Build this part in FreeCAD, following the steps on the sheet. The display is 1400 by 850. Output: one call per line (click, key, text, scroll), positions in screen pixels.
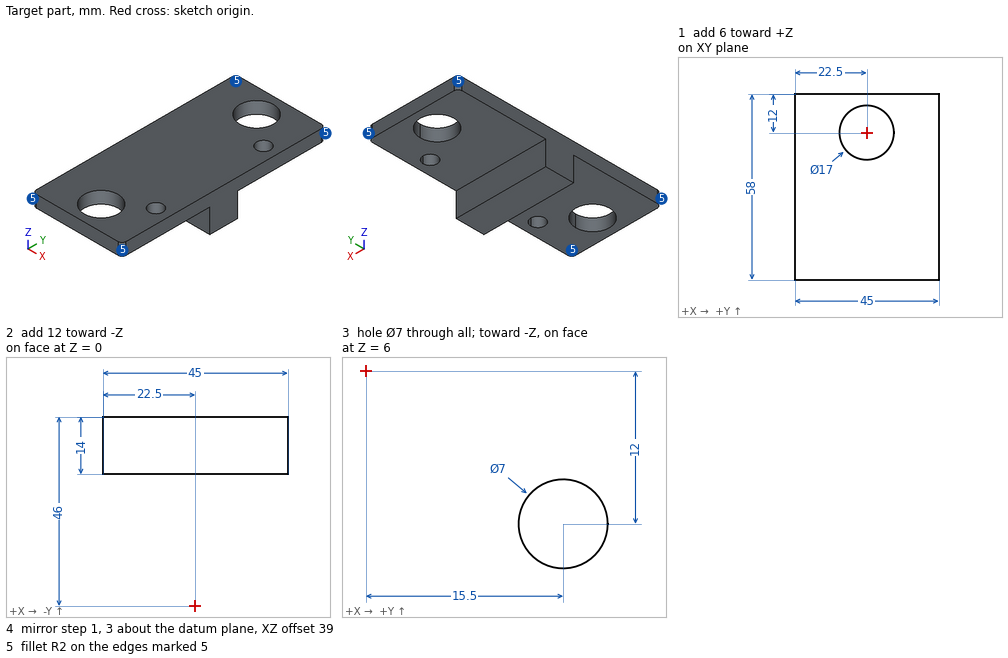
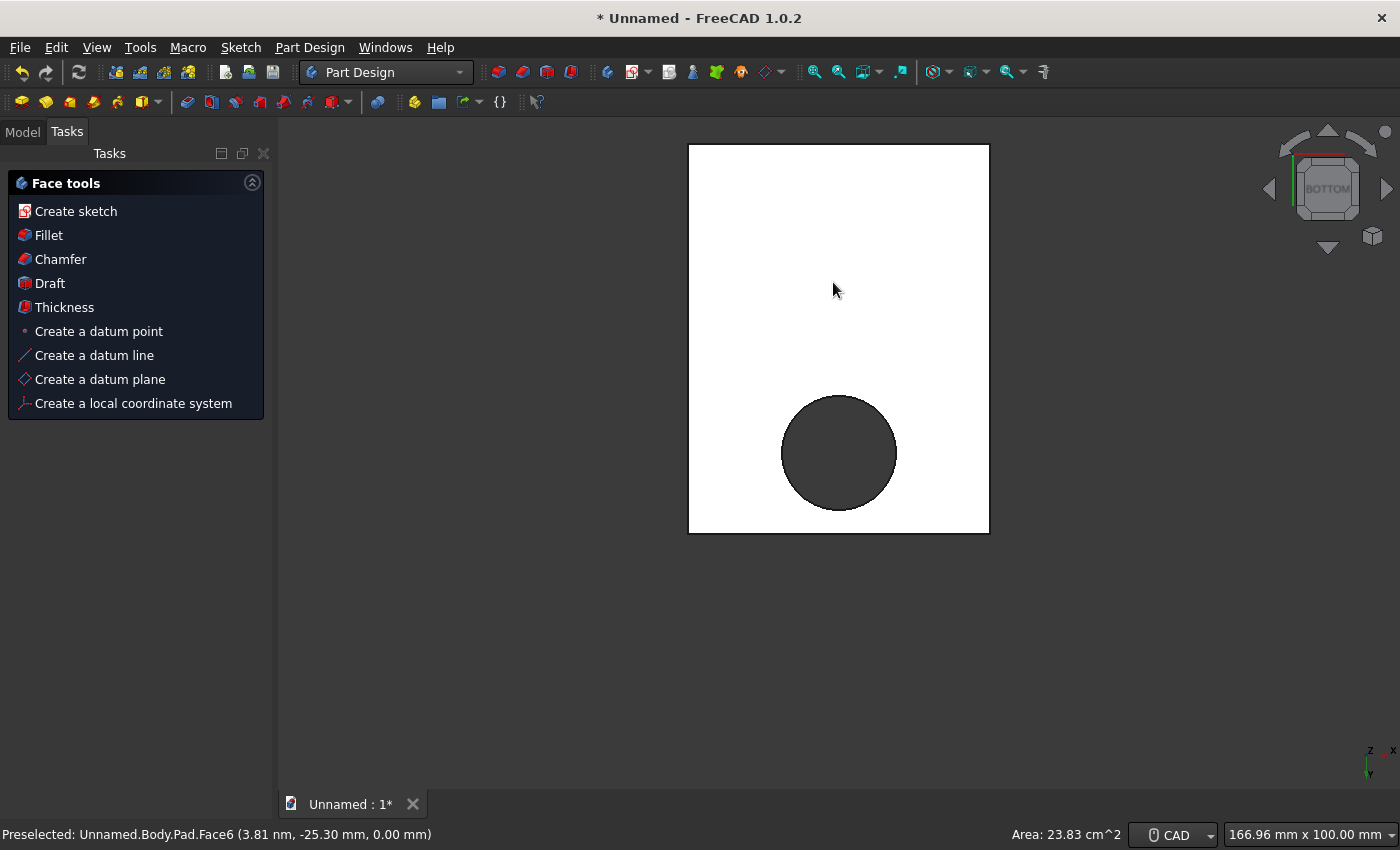
click(632, 72)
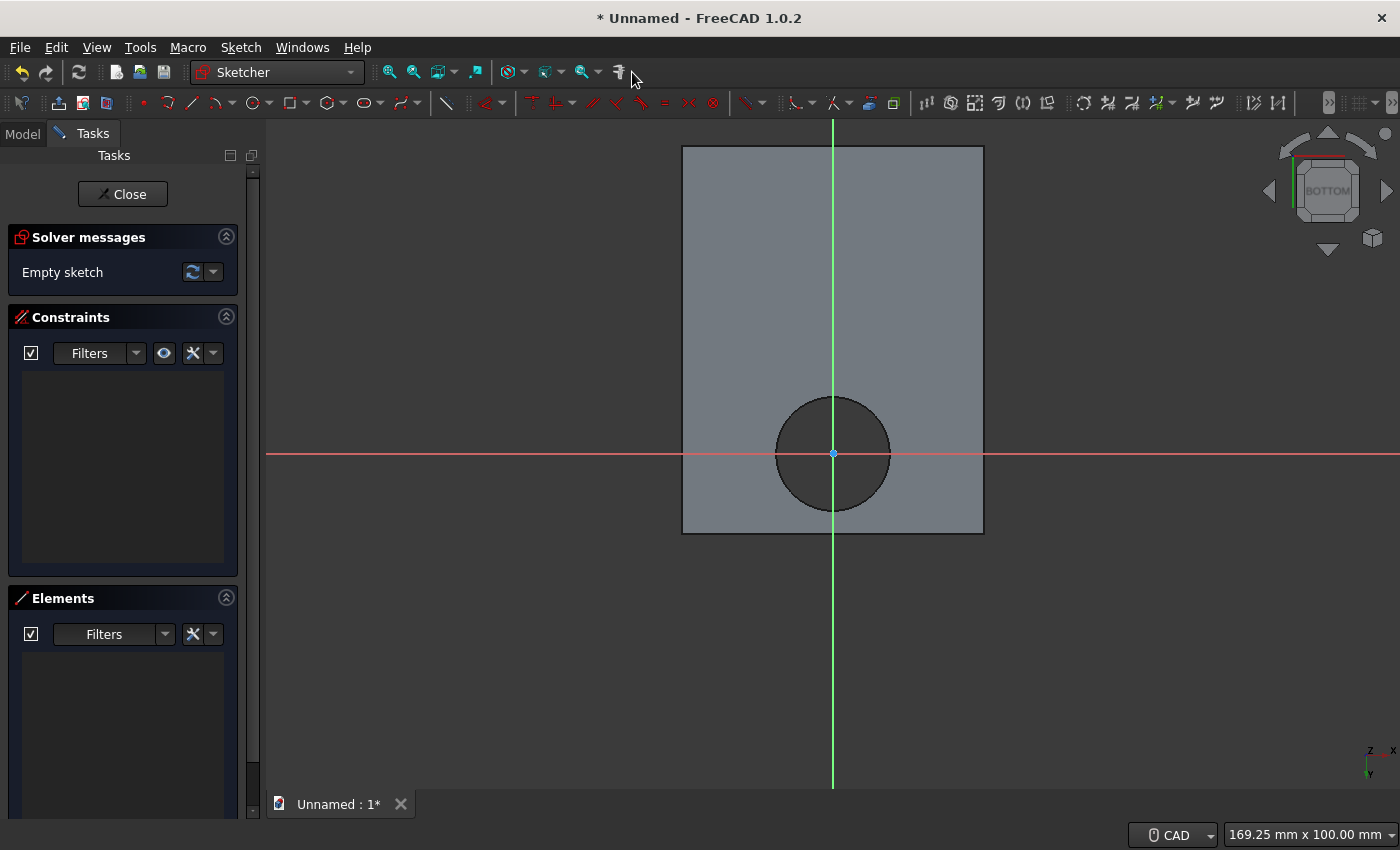
scroll(455, 761, down, 1)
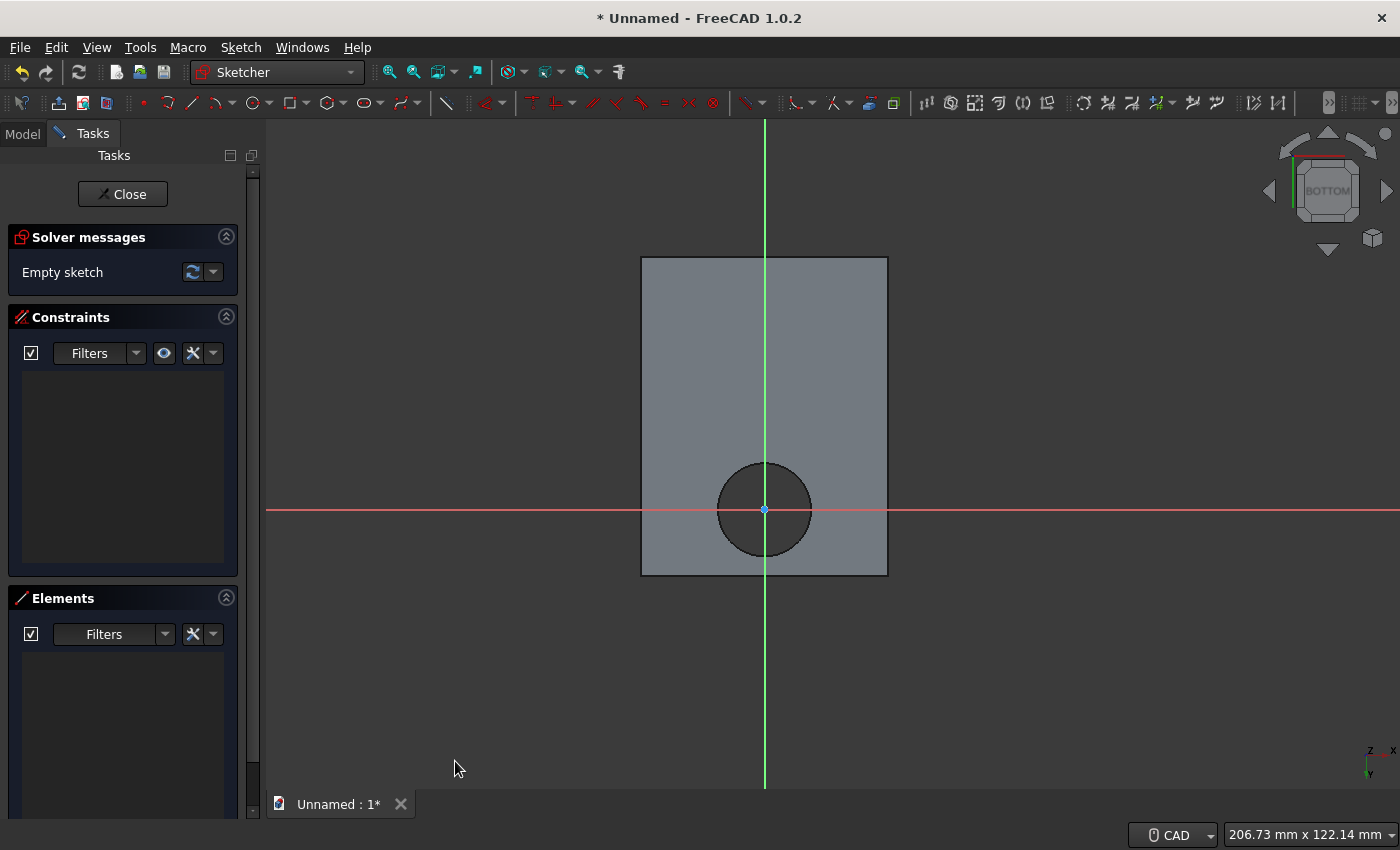
scroll(765, 298, up, 3)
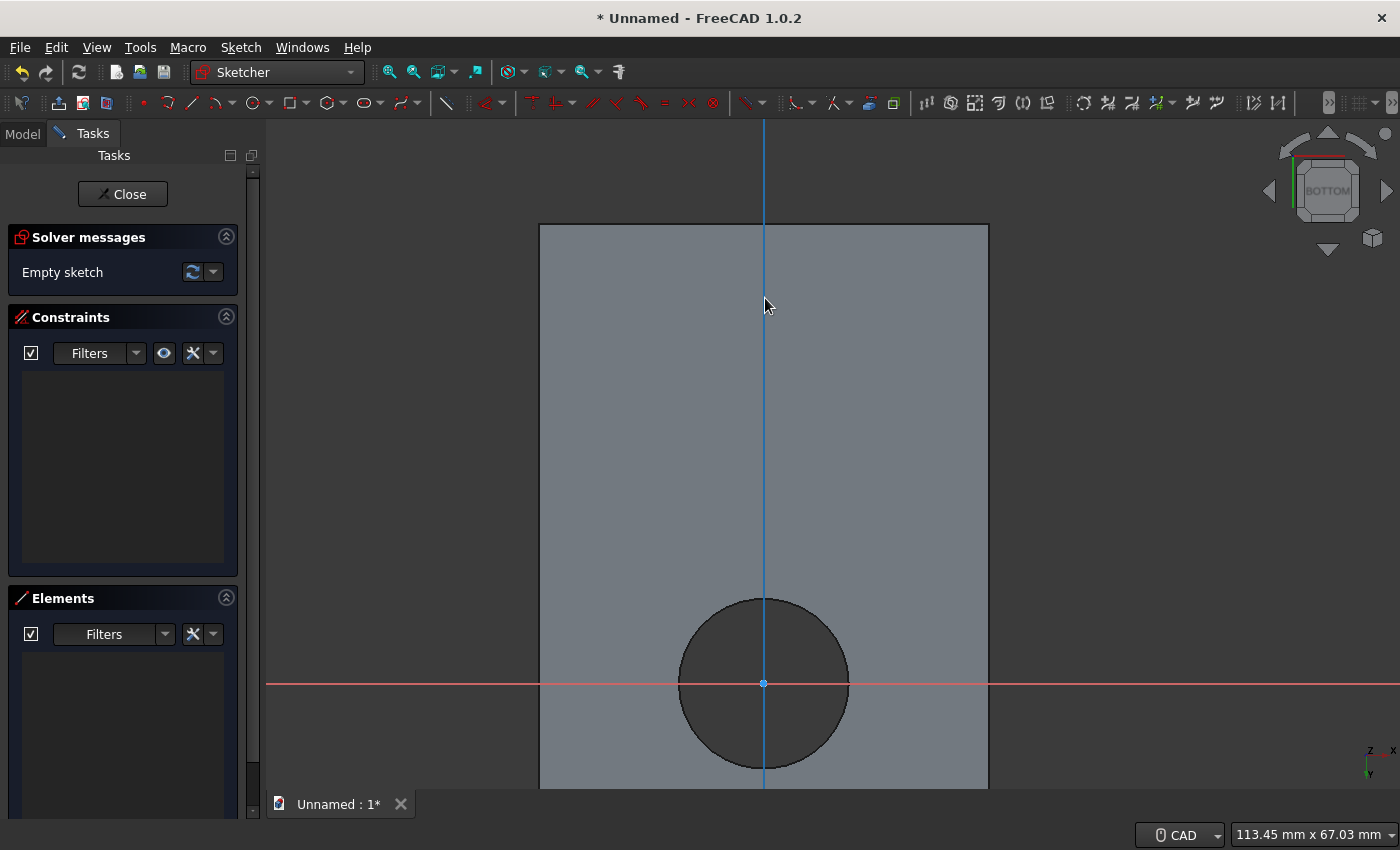
click(290, 104)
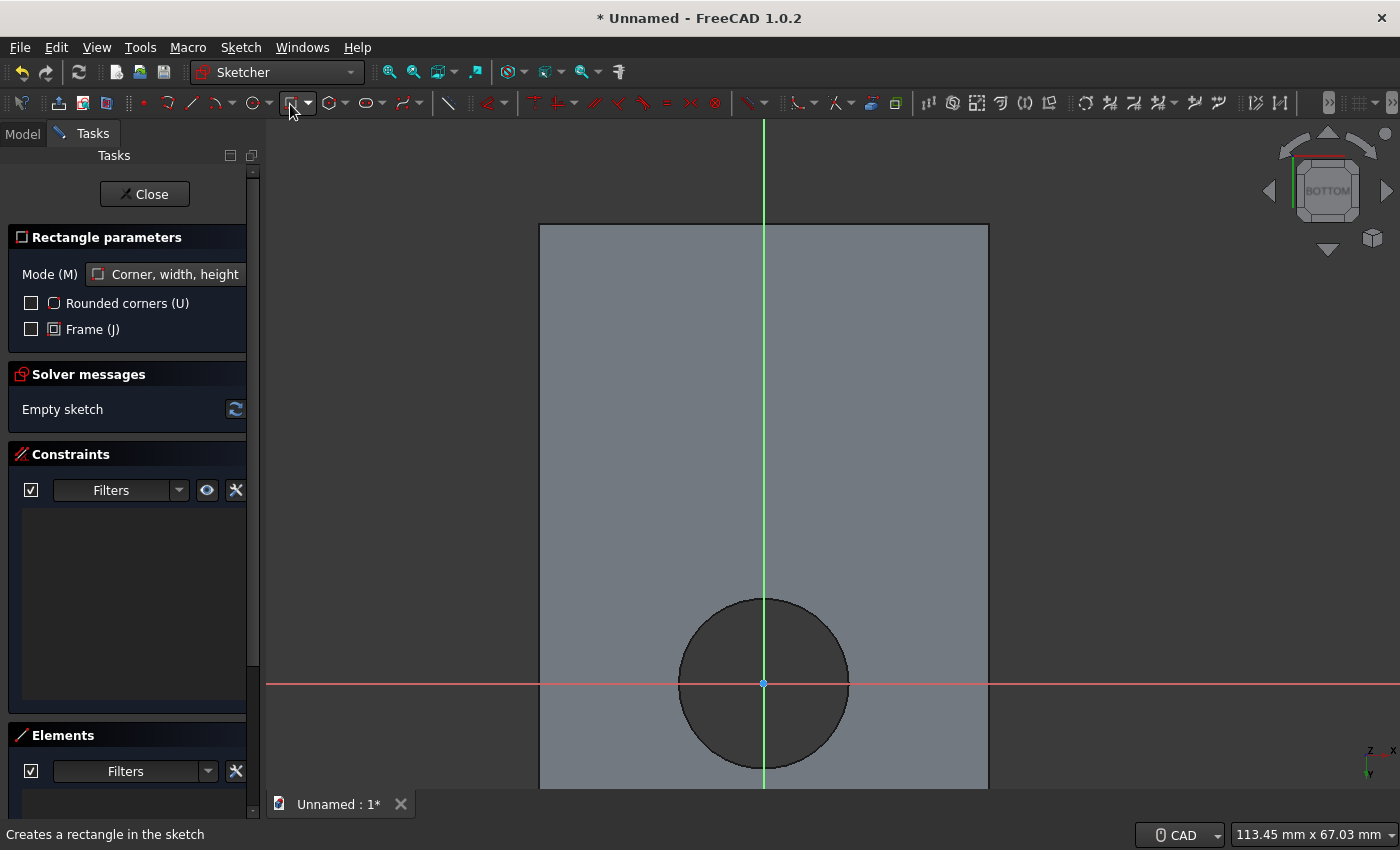
click(539, 224)
click(989, 364)
key(Escape)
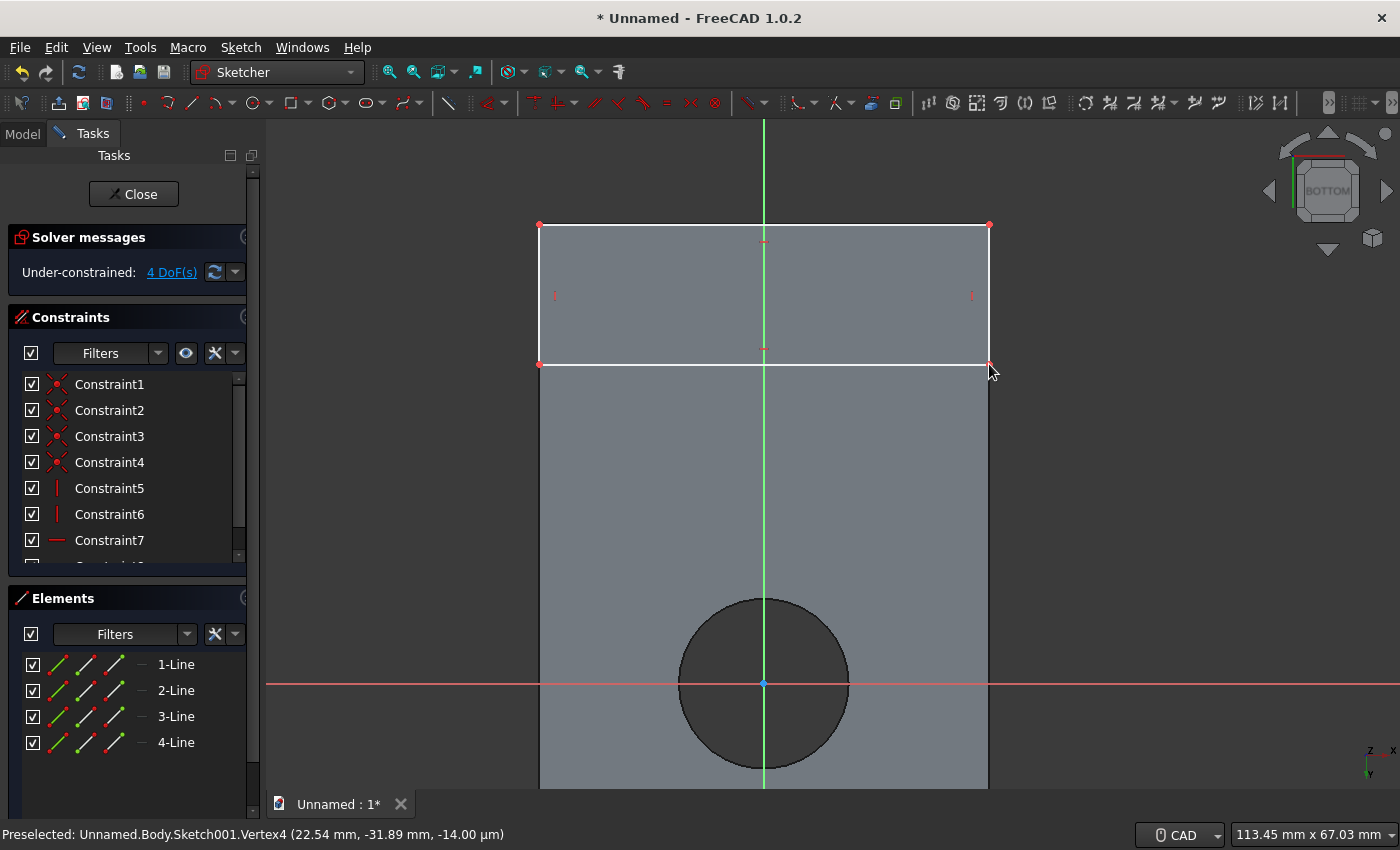
click(488, 104)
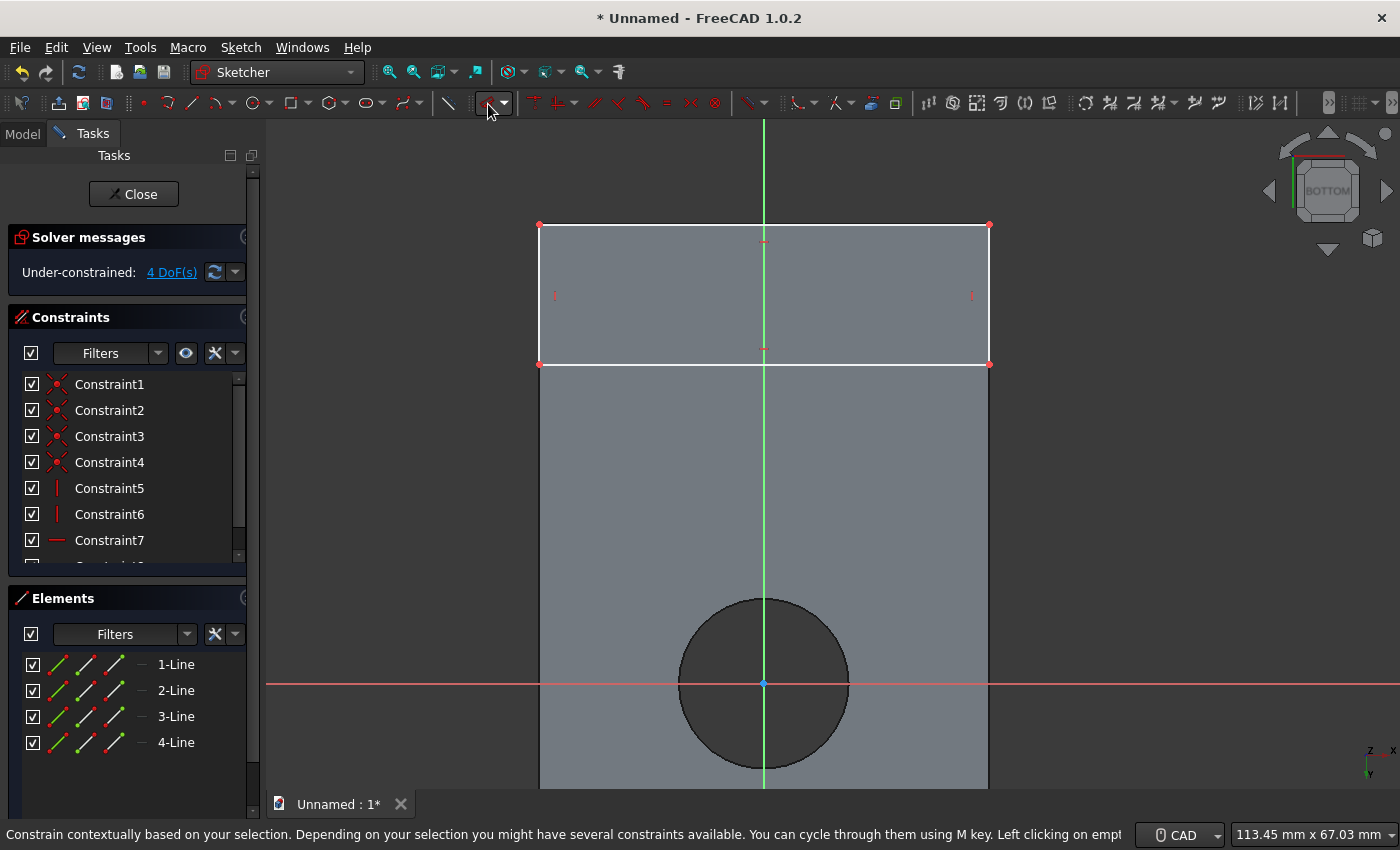
click(539, 267)
click(505, 295)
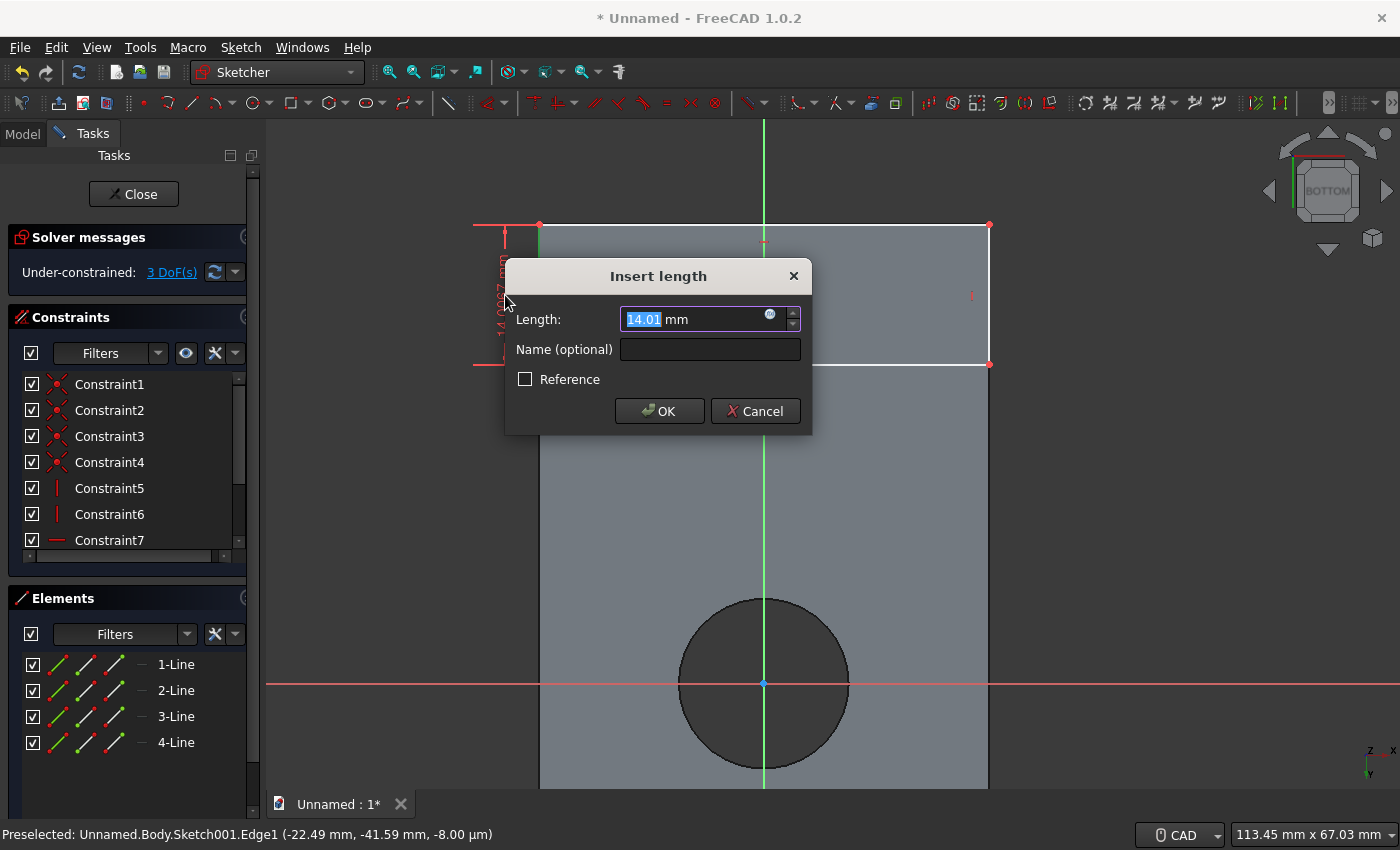
text(14)
key(Return)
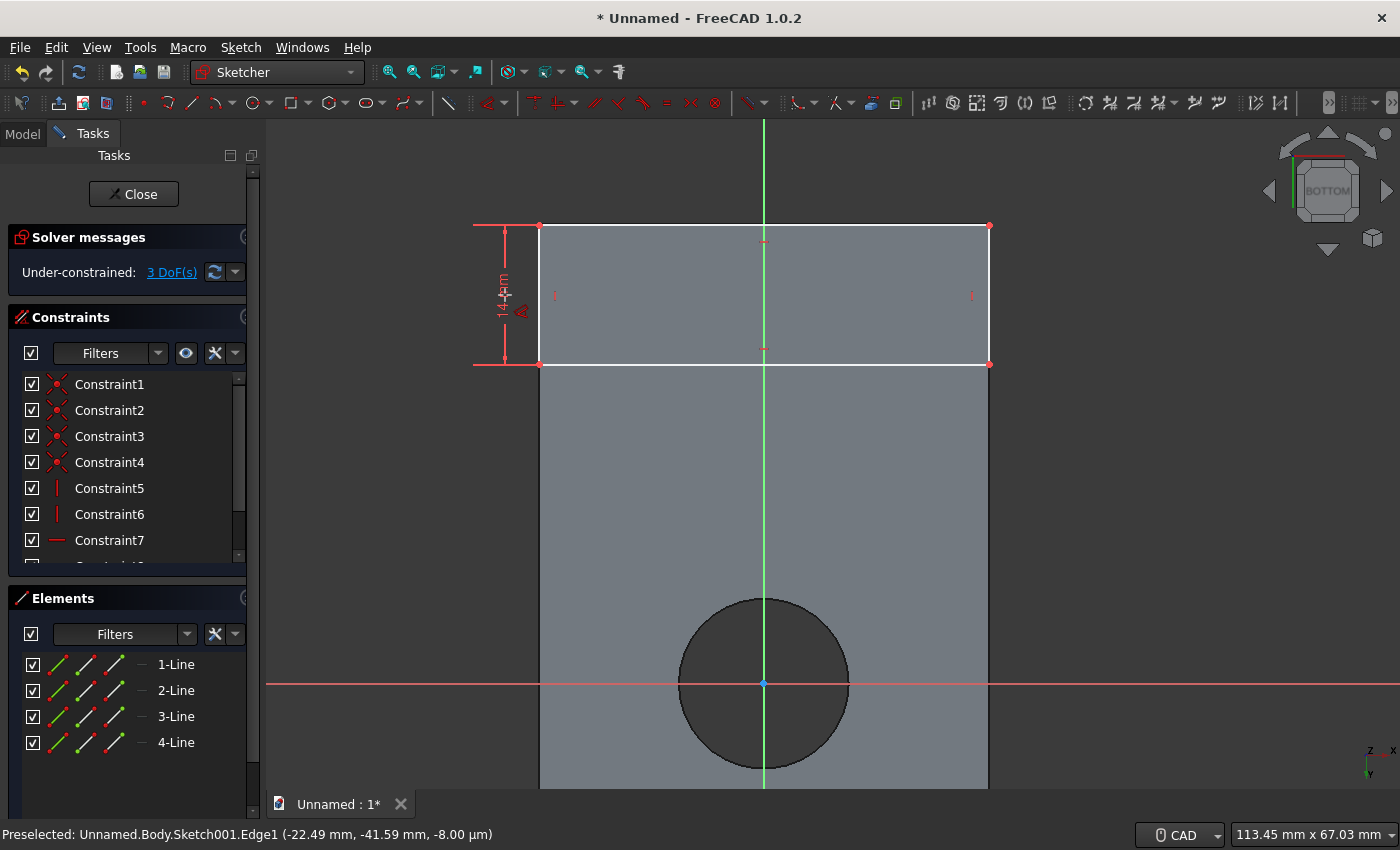
click(674, 365)
click(661, 331)